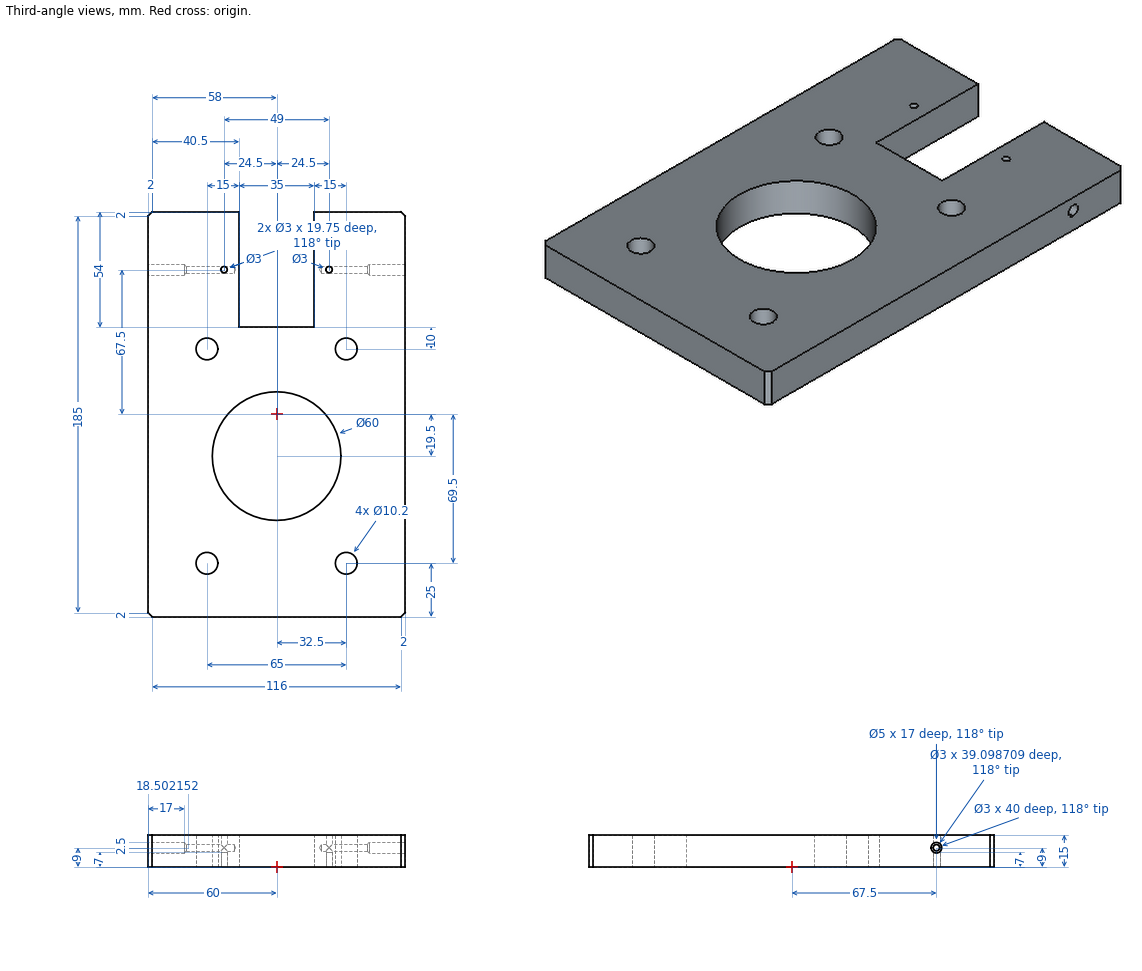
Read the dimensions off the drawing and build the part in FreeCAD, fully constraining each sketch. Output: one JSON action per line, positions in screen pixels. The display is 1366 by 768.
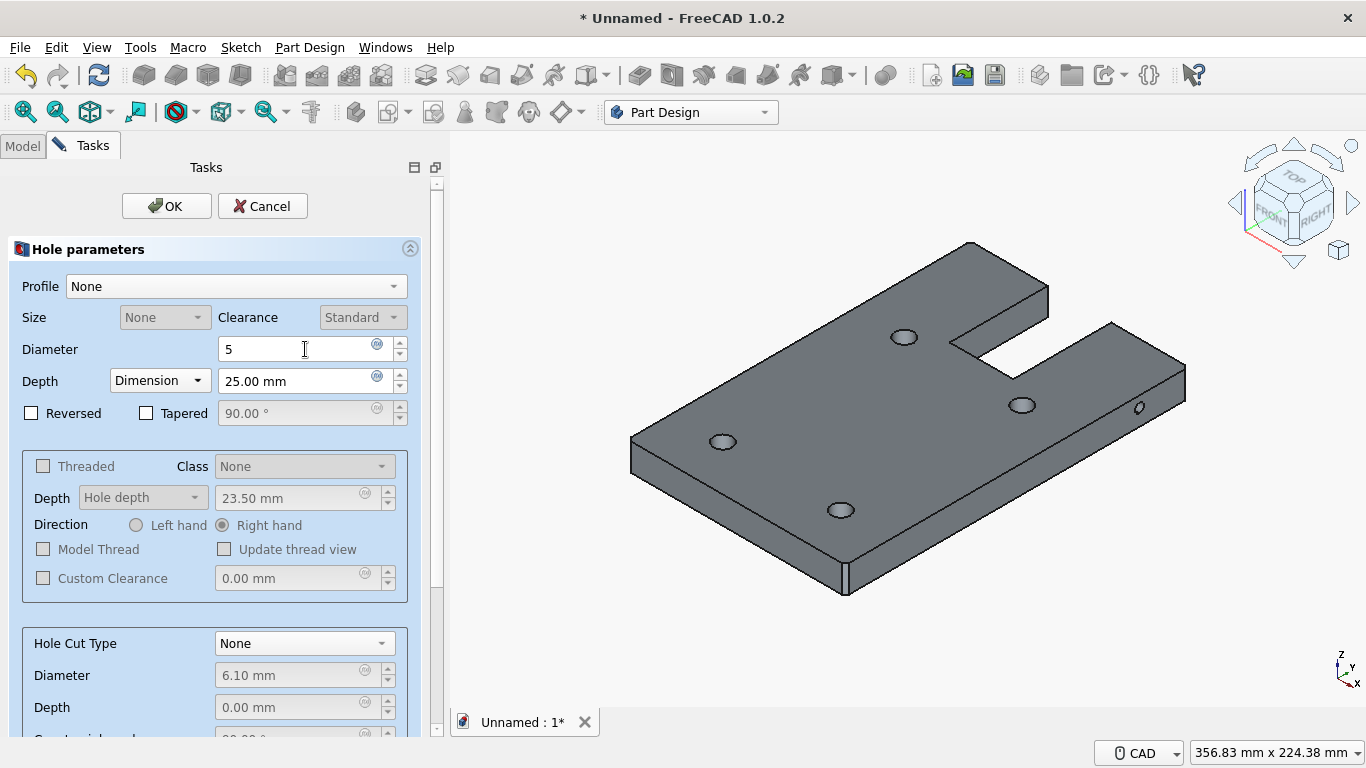
{"action": "triple_click", "coordinate": [305, 381]}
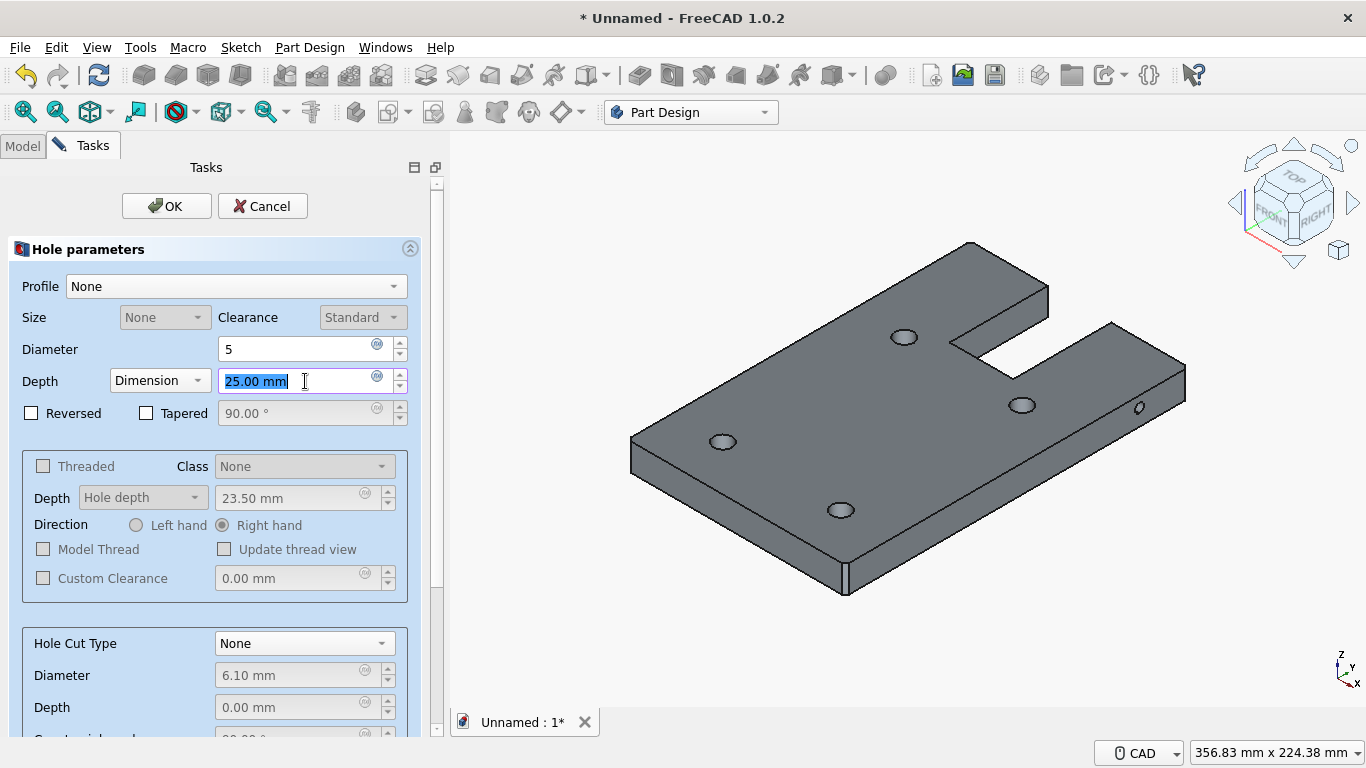
{"action": "type", "text": "17"}
{"action": "key", "text": "Tab"}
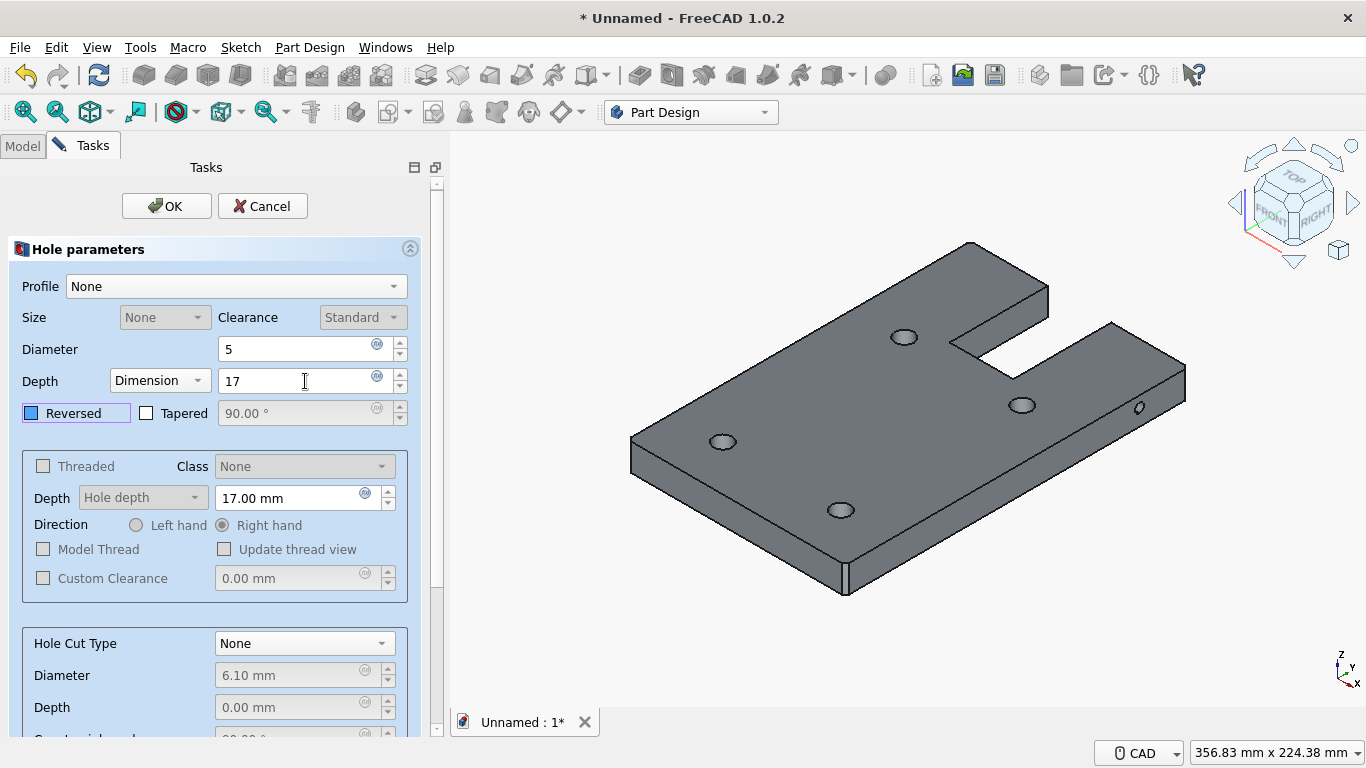
{"action": "left_click", "coordinate": [167, 206]}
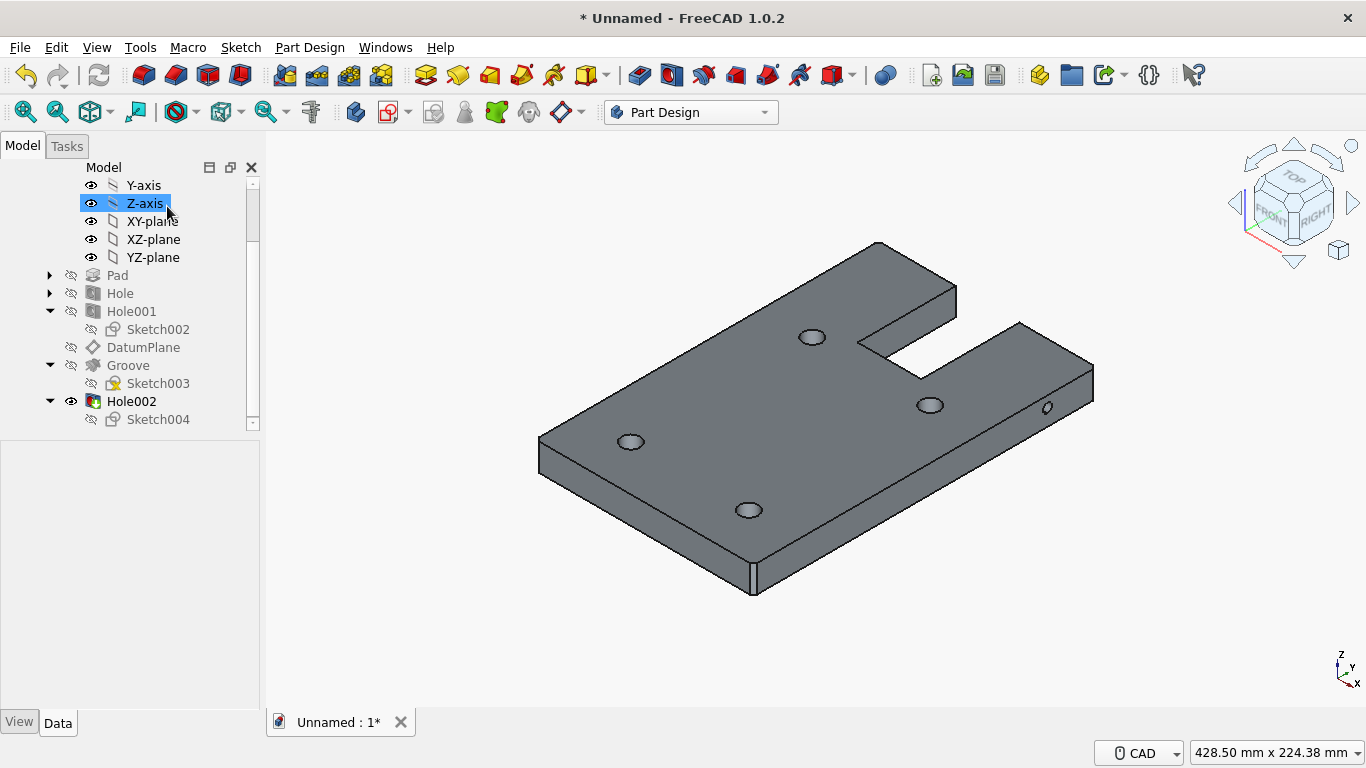
{"action": "left_click", "coordinate": [767, 431]}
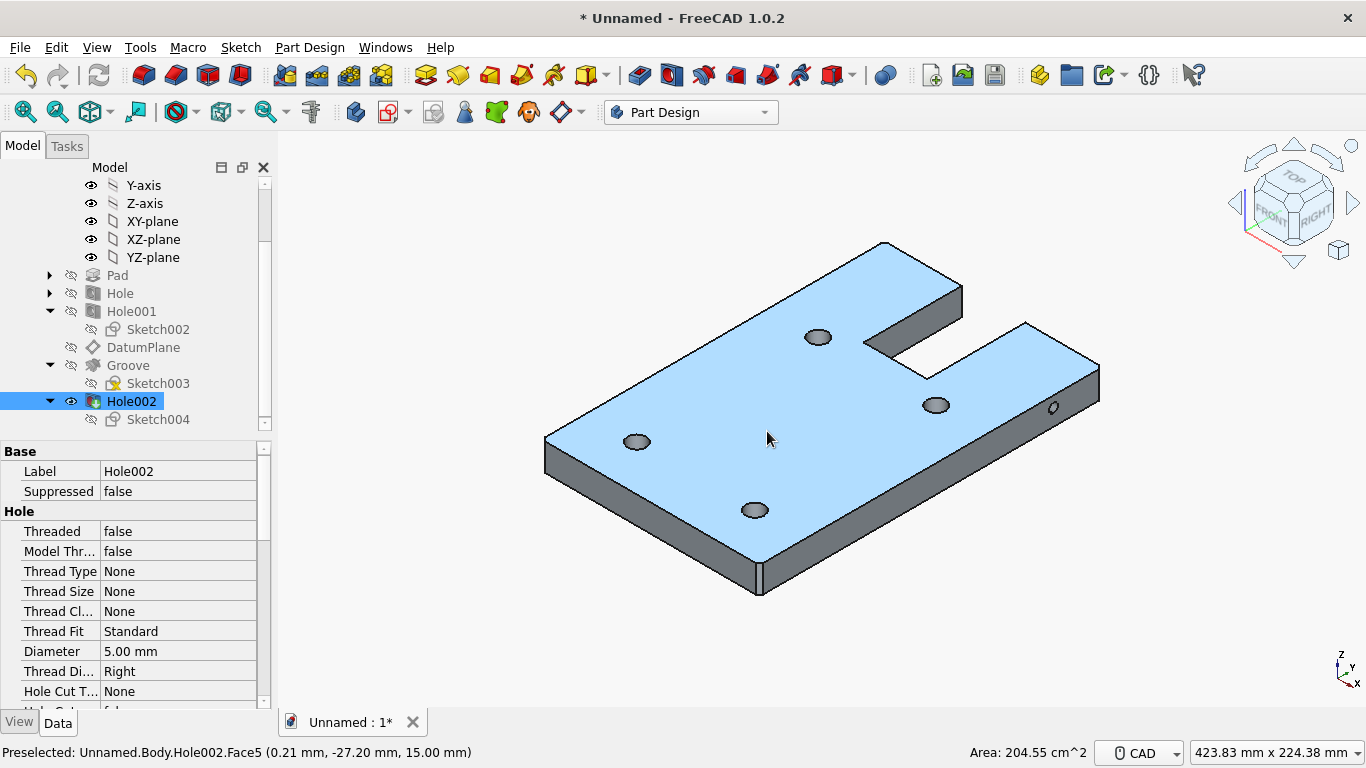
{"action": "left_click", "coordinate": [388, 112]}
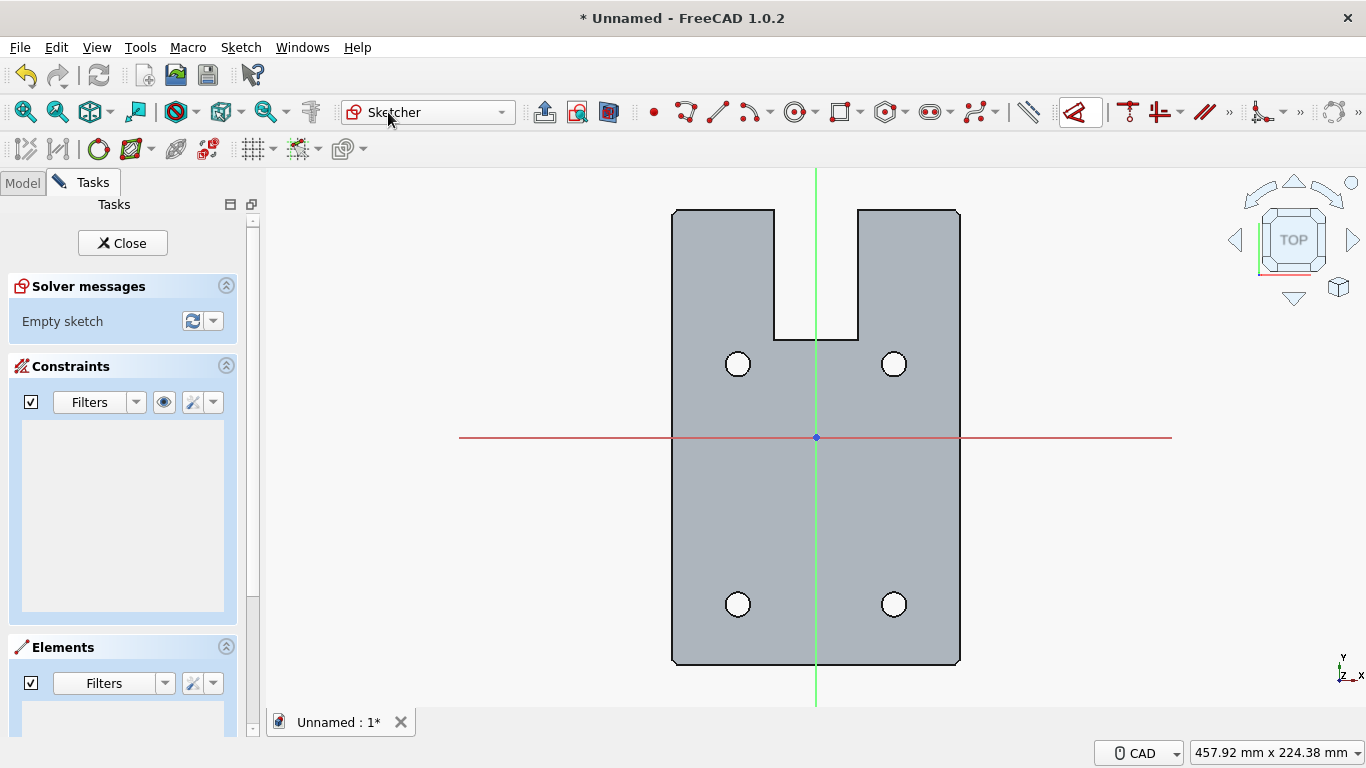
{"action": "scroll", "coordinate": [872, 523], "scroll_direction": "up", "scroll_amount": 4}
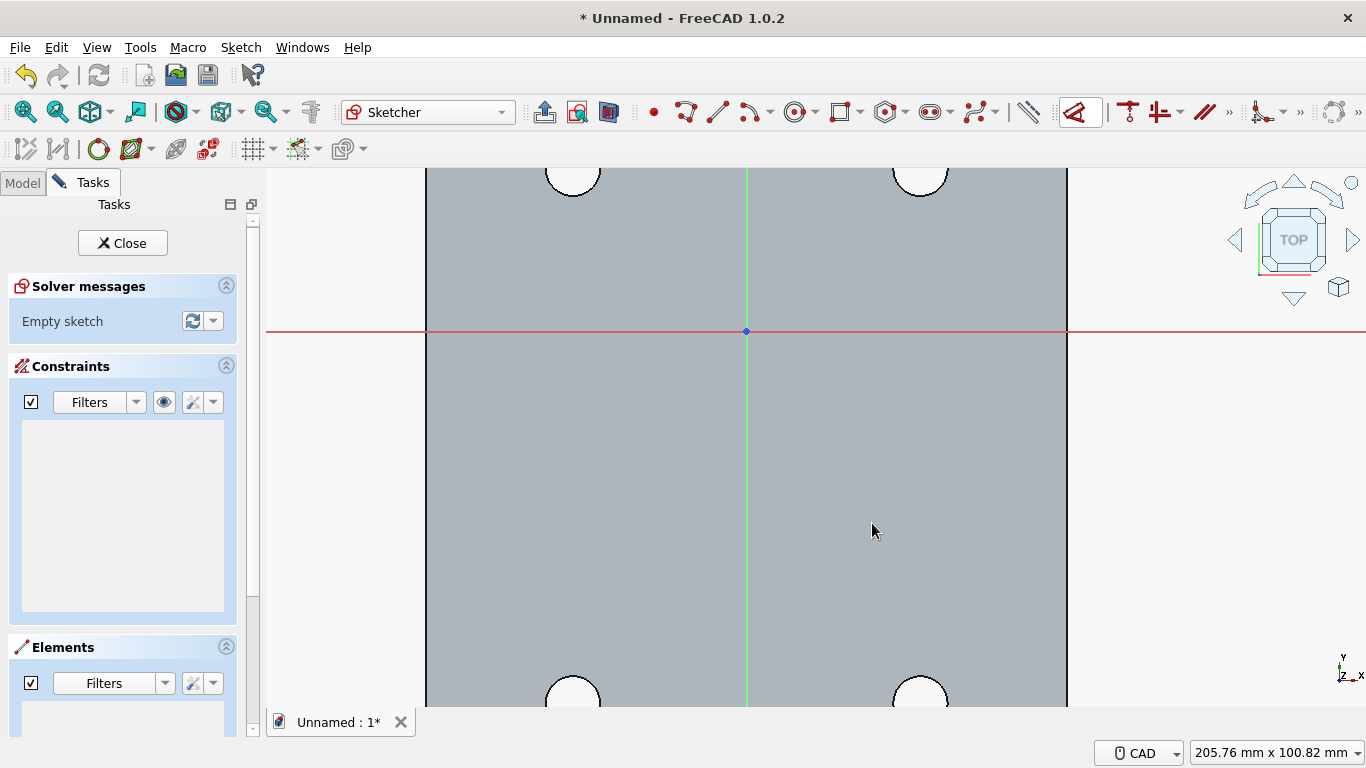
{"action": "key", "text": "g c"}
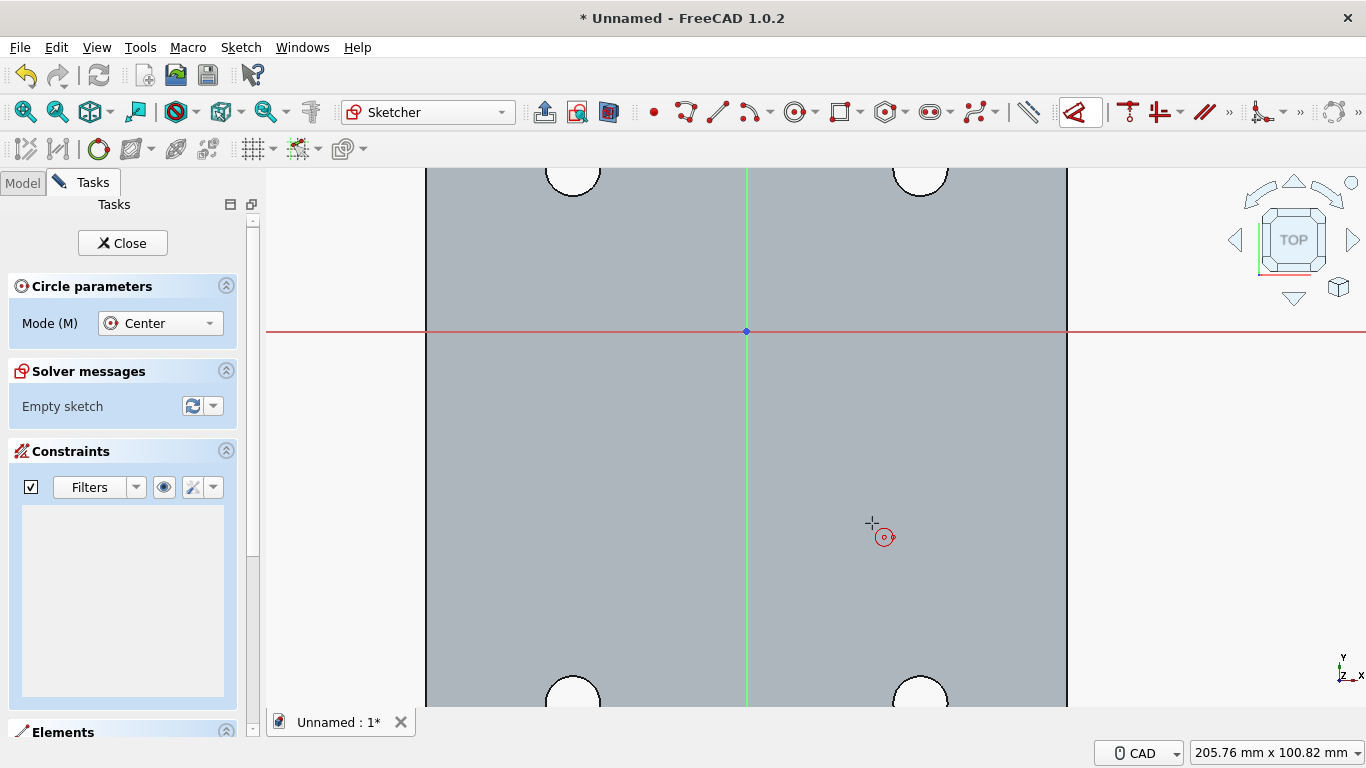
{"action": "left_click", "coordinate": [747, 436]}
{"action": "mouse_move", "coordinate": [860, 550]}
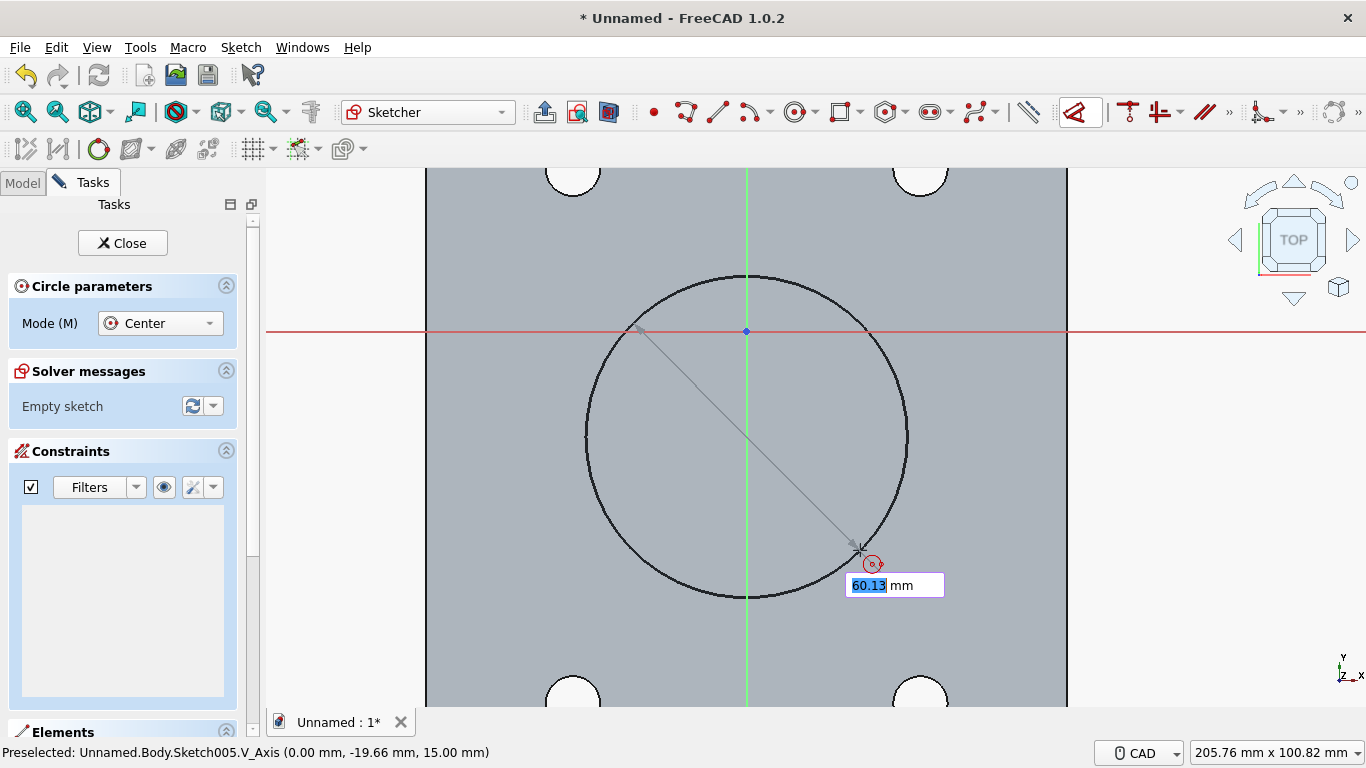
{"action": "type", "text": "60"}
{"action": "key", "text": "Return"}
{"action": "key", "text": "Escape"}